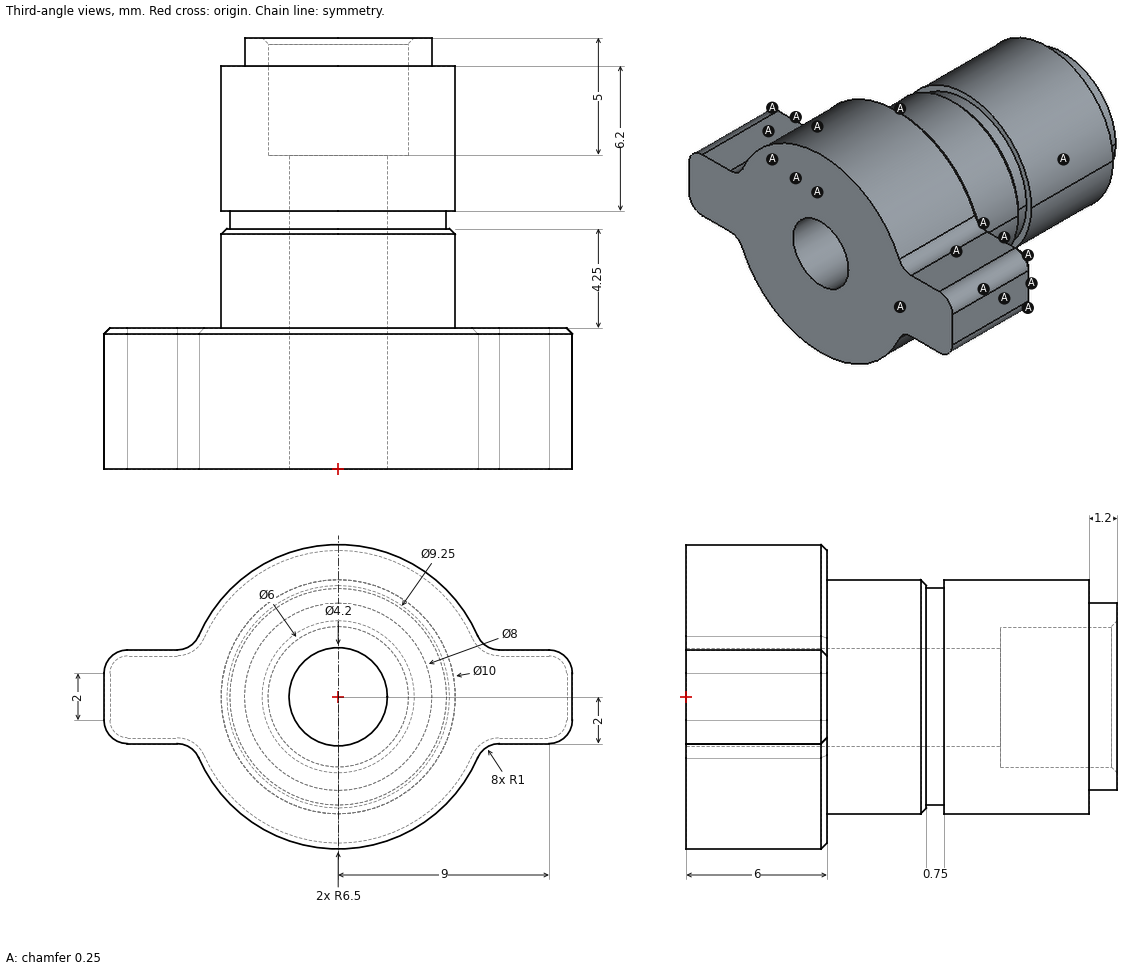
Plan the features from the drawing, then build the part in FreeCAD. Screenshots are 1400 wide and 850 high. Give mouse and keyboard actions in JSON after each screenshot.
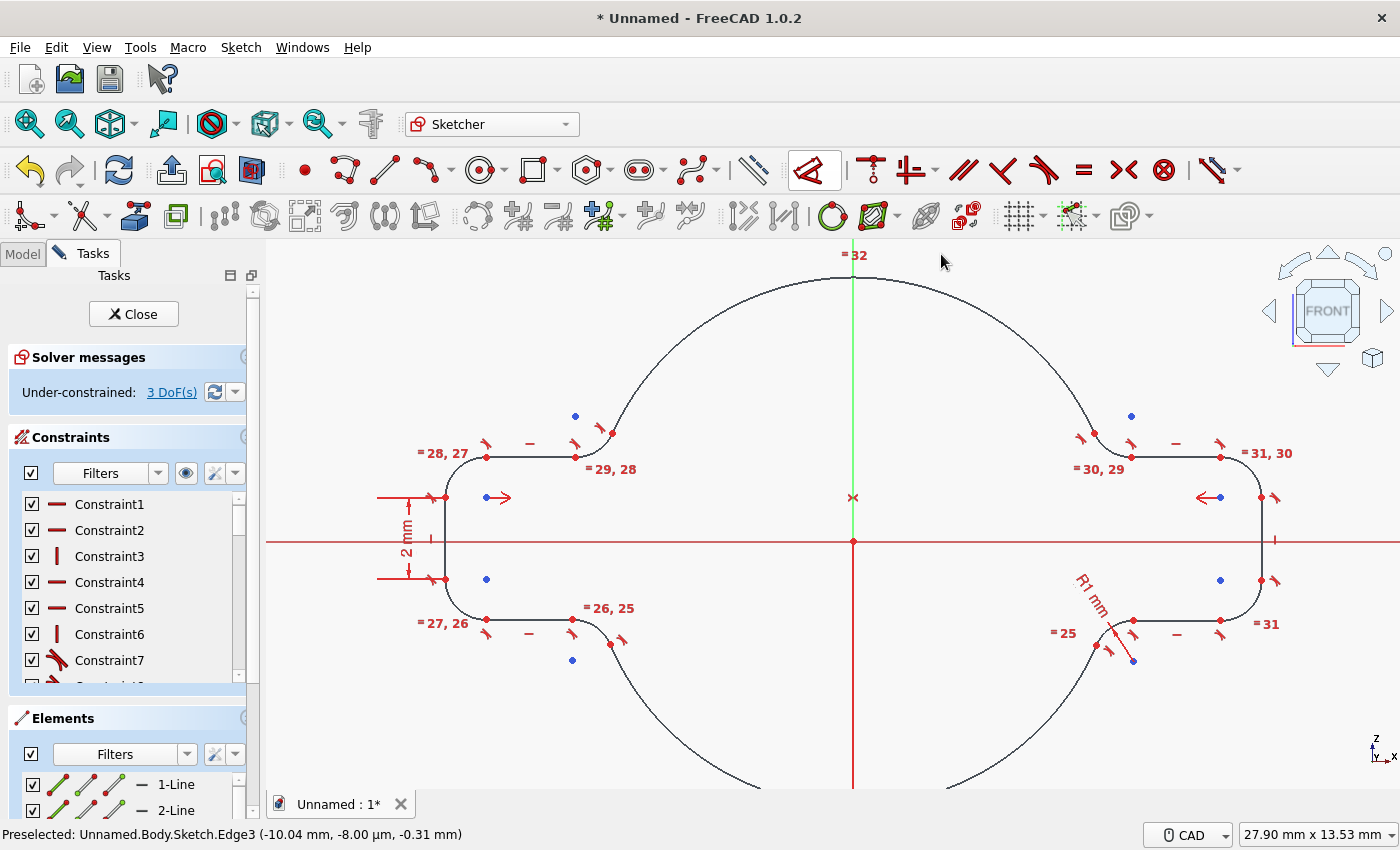
{"action": "scroll", "coordinate": [584, 458], "scroll_direction": "down", "scroll_amount": 2}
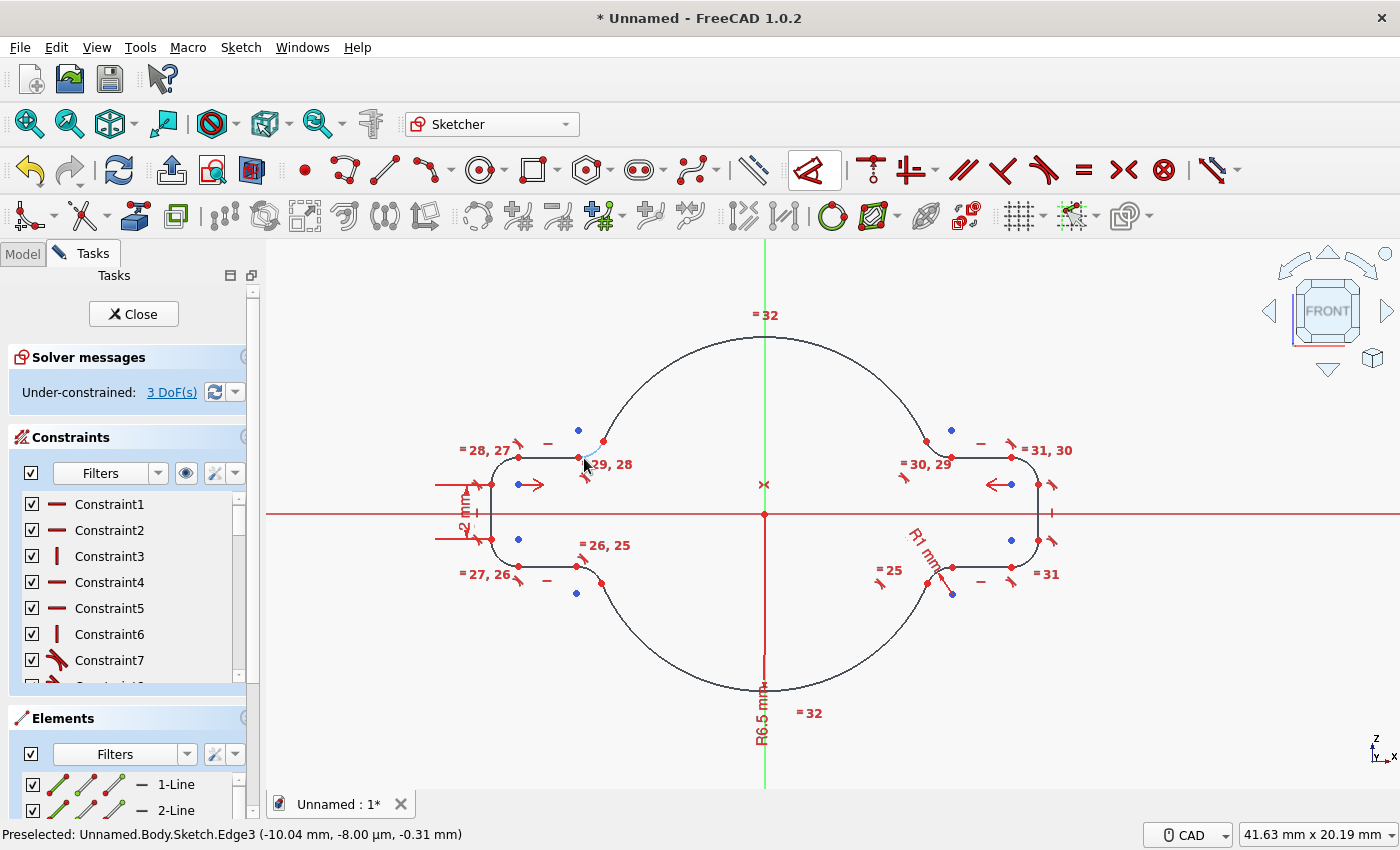
{"action": "left_click", "coordinate": [1038, 501]}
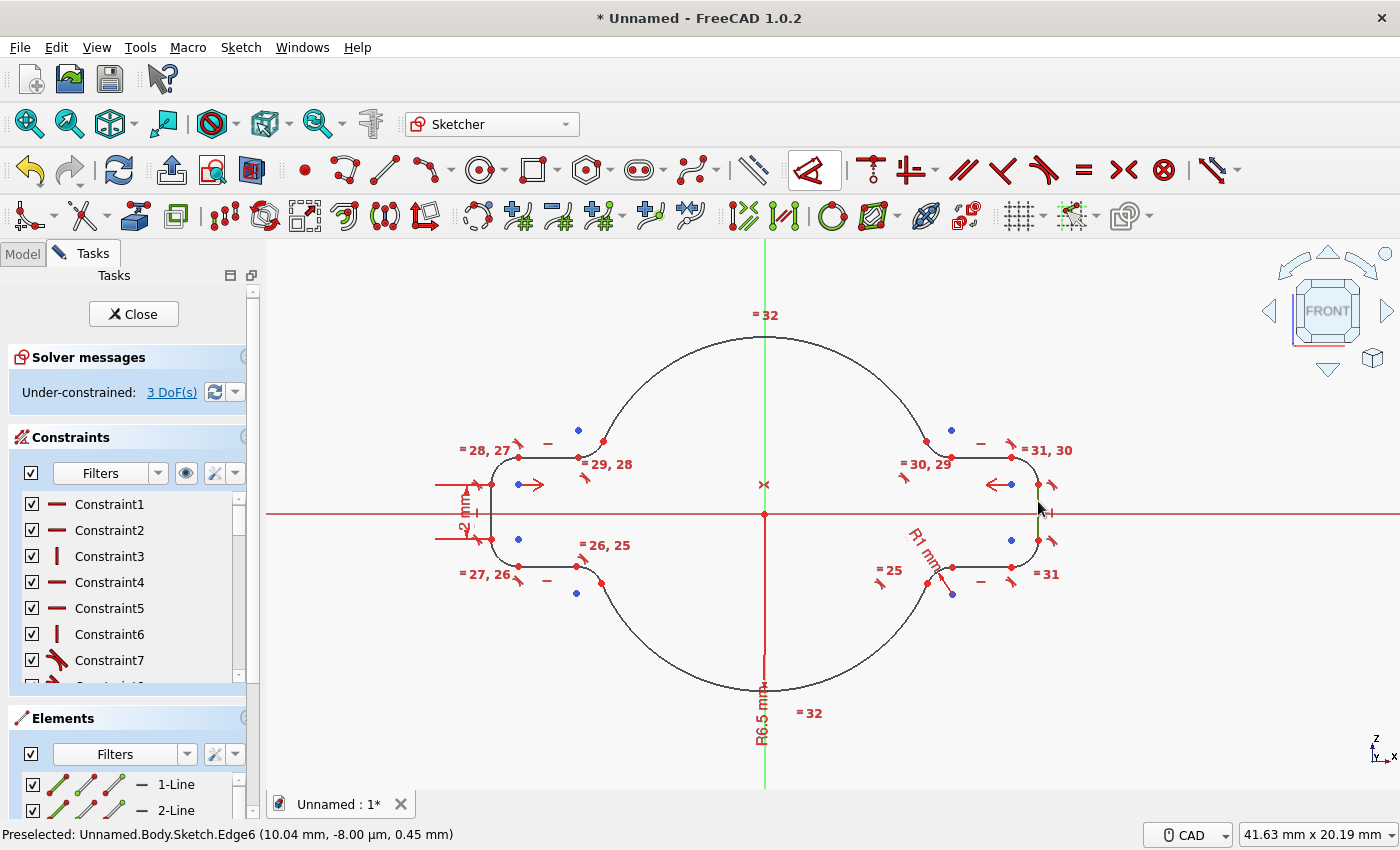
{"action": "key", "text": "i"}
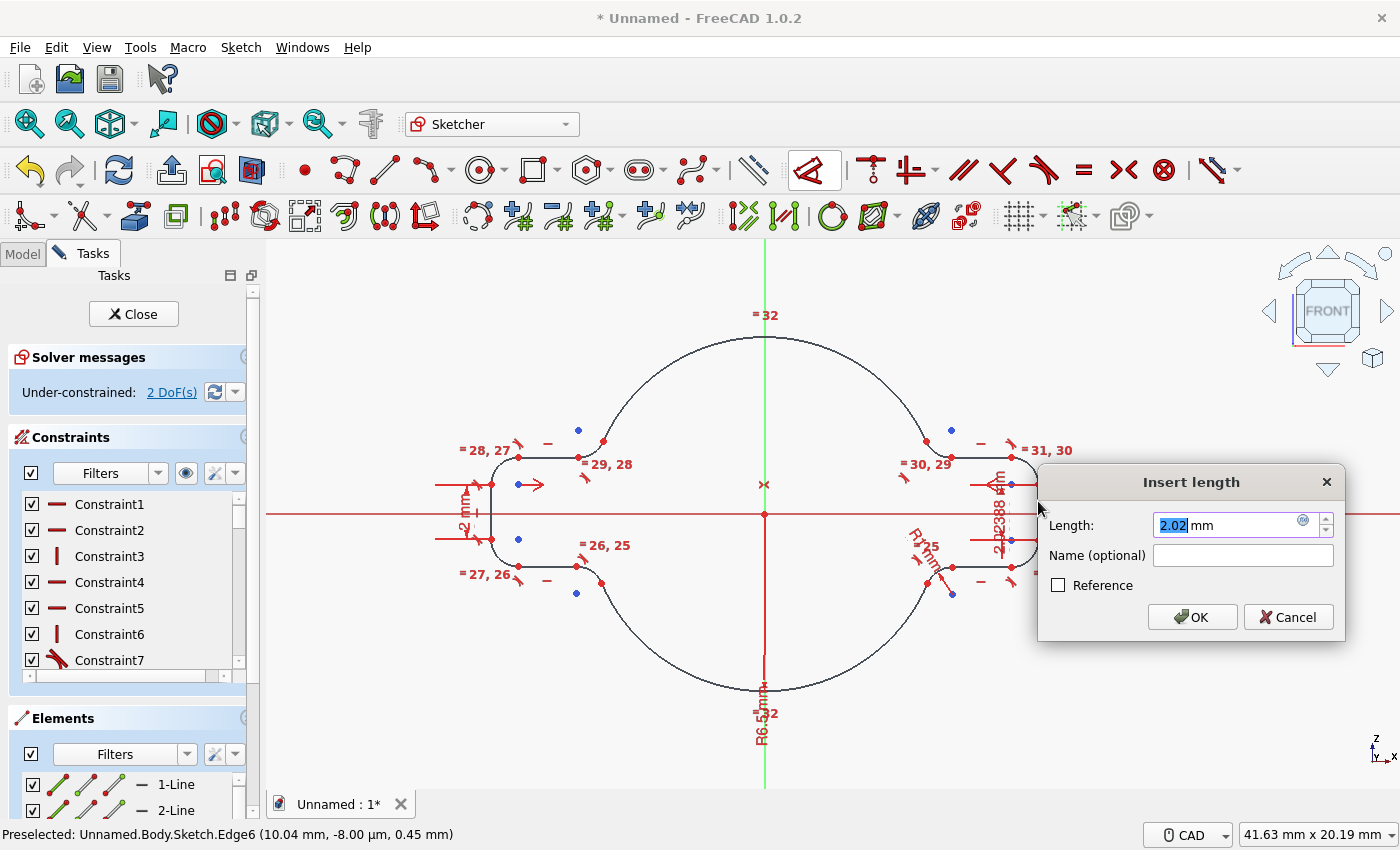
{"action": "type", "text": "2"}
{"action": "key", "text": "Return"}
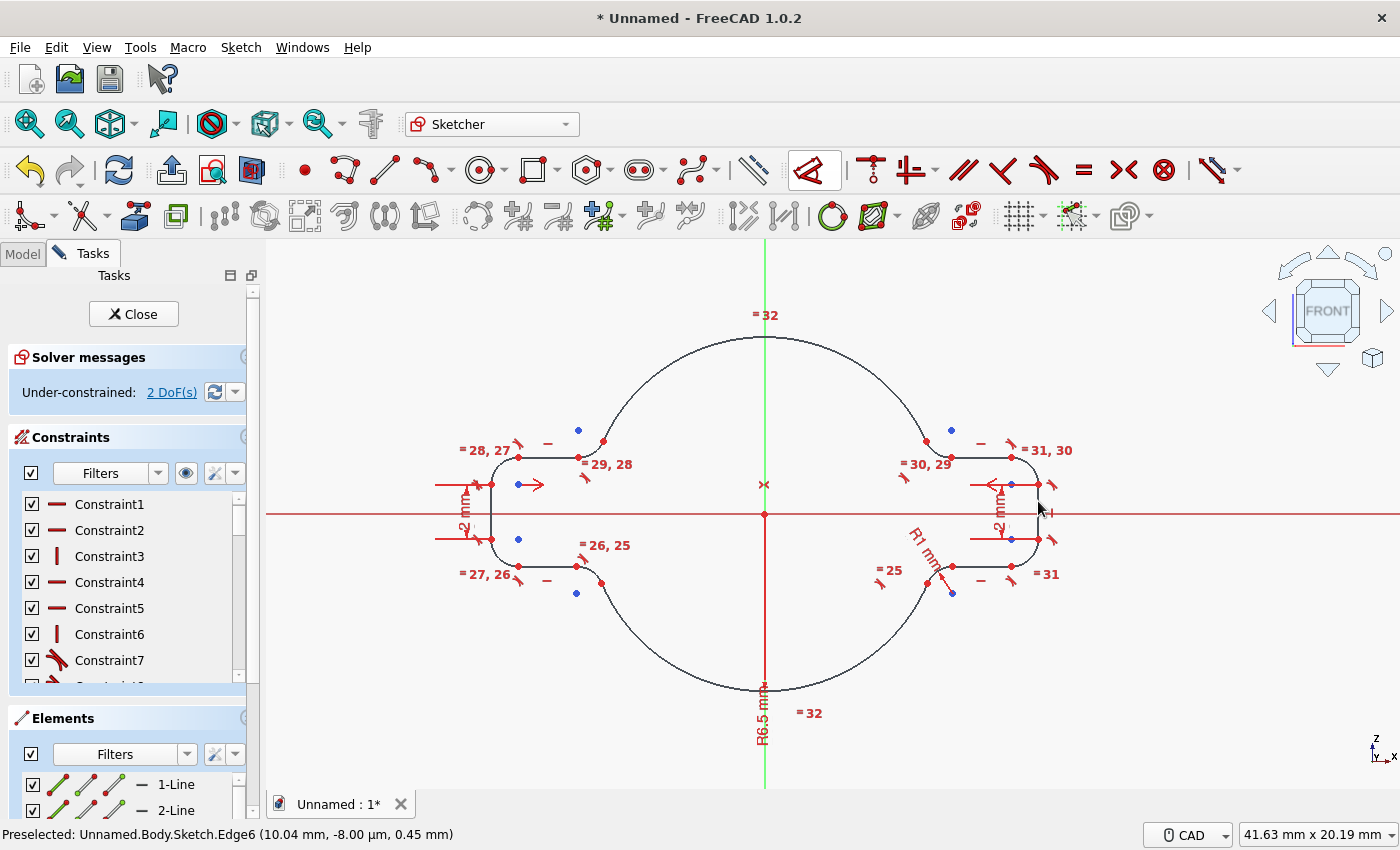
{"action": "left_click", "coordinate": [1011, 567]}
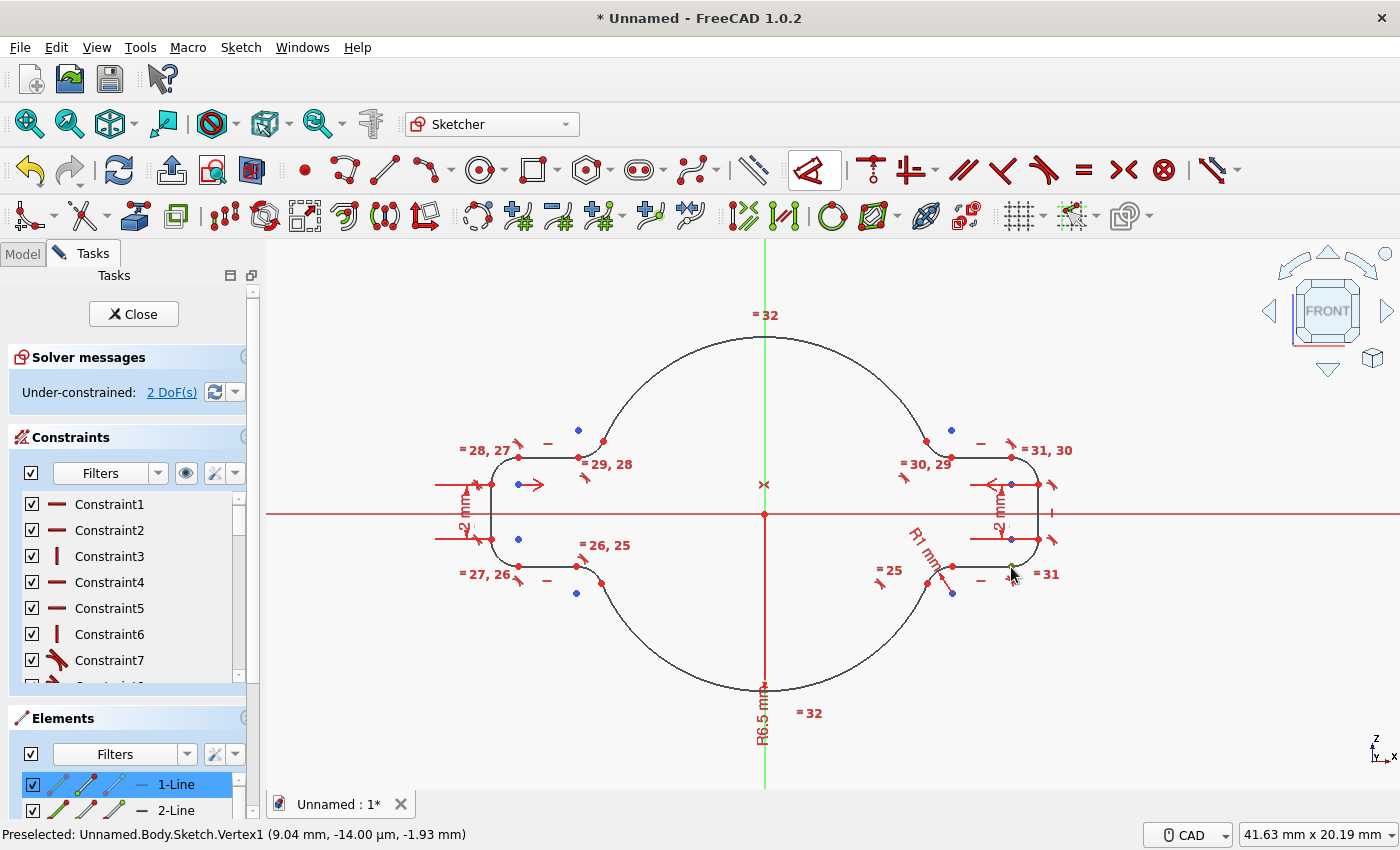
{"action": "left_click", "coordinate": [836, 170]}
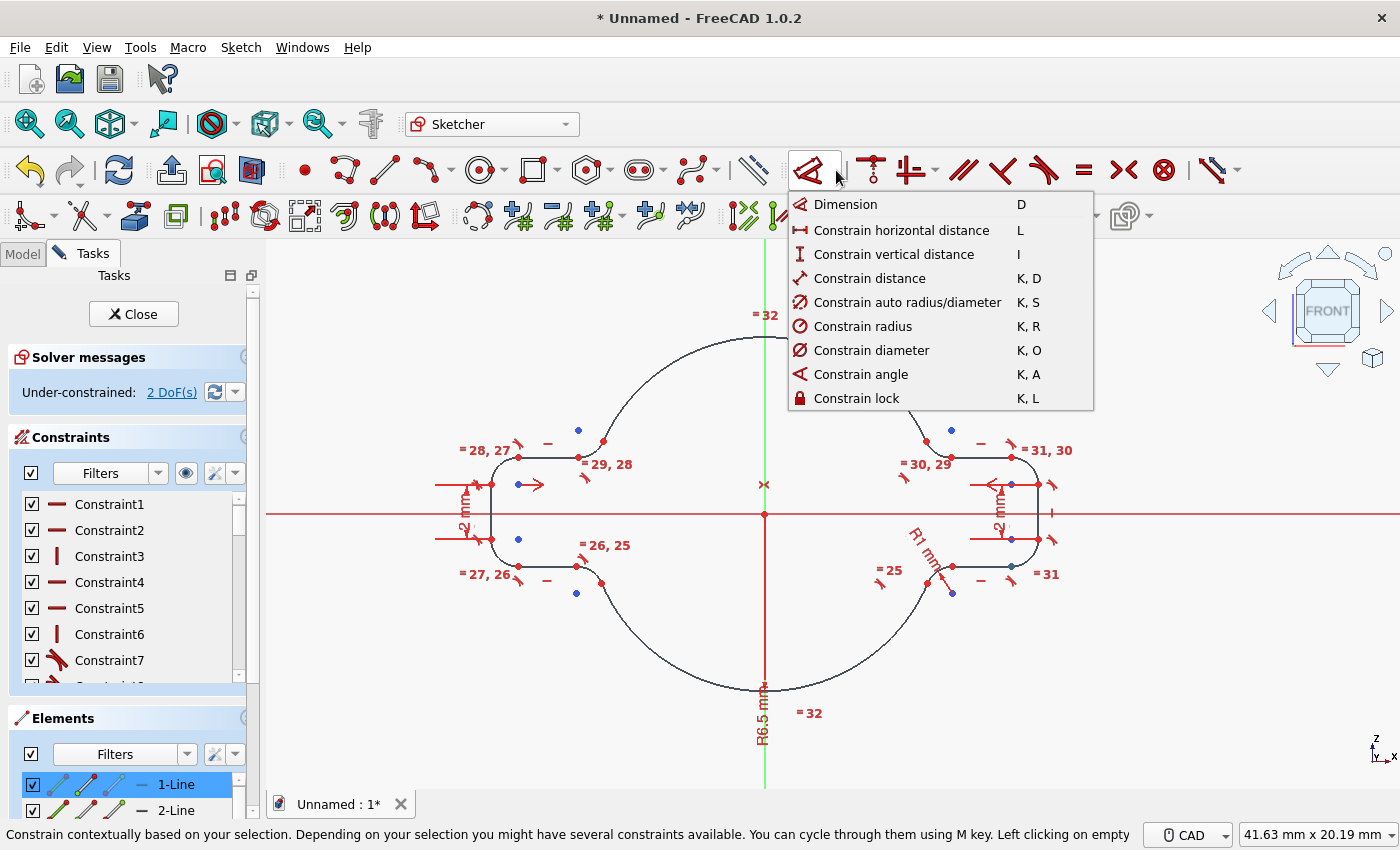
{"action": "left_click", "coordinate": [941, 230]}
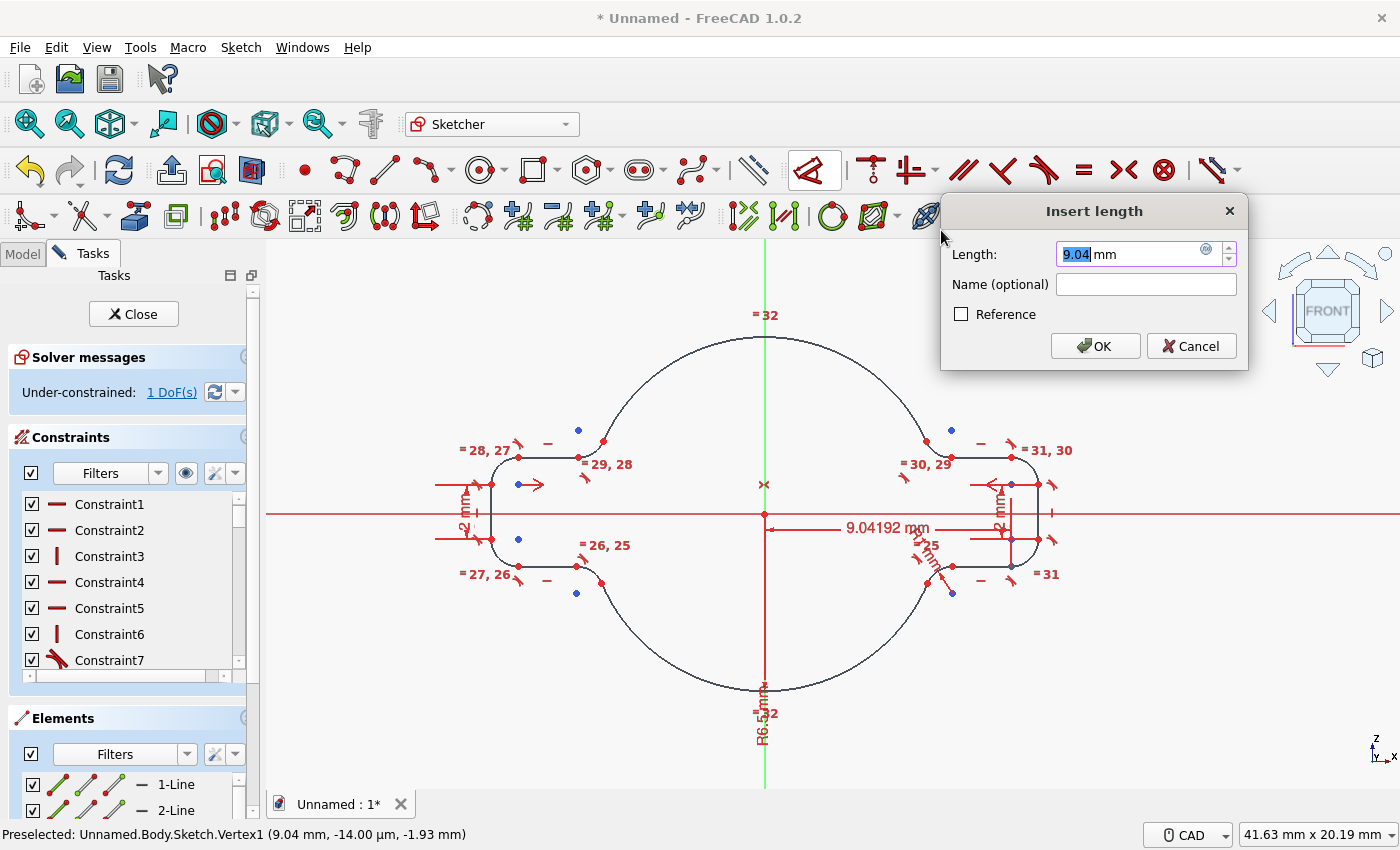
{"action": "type", "text": "9"}
{"action": "key", "text": "Return"}